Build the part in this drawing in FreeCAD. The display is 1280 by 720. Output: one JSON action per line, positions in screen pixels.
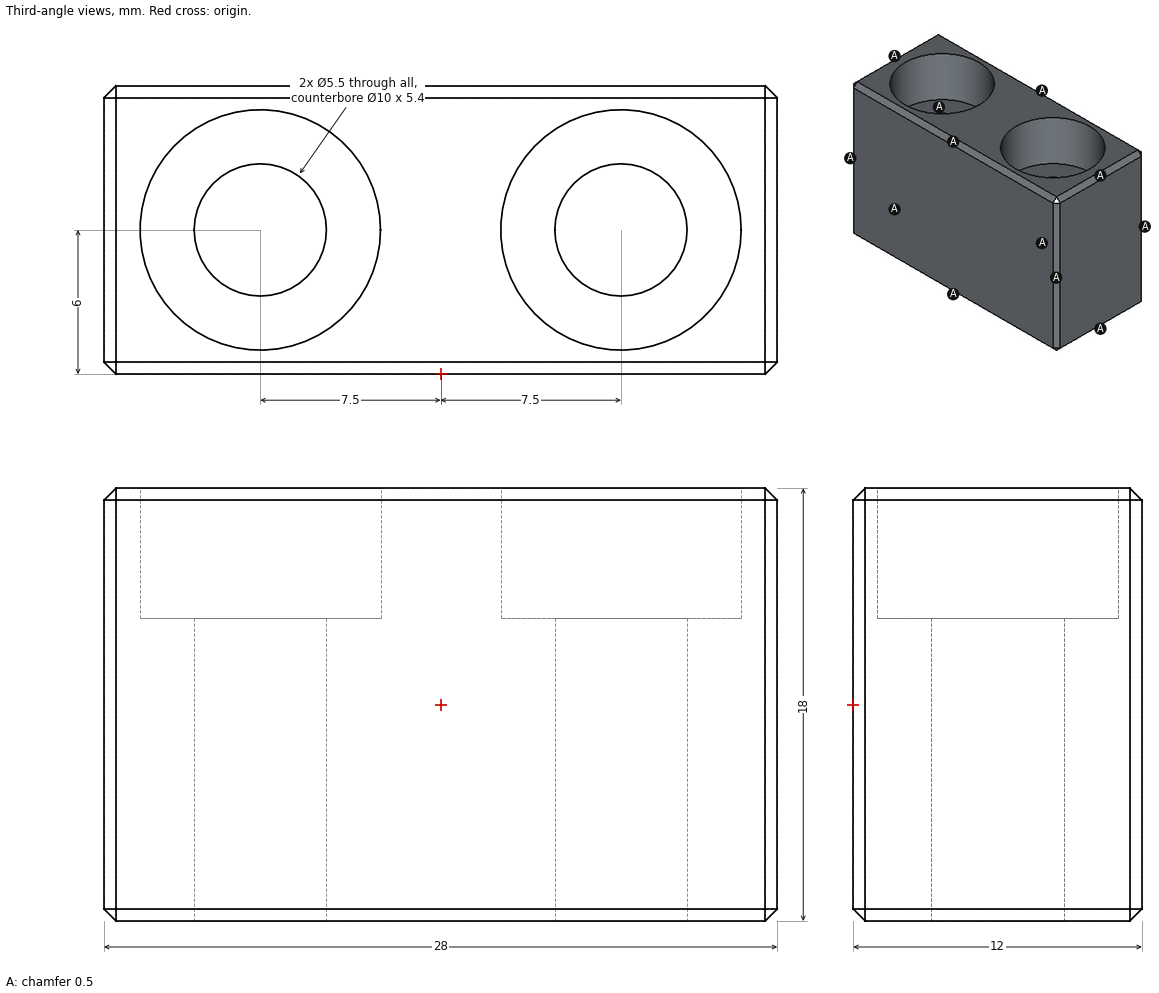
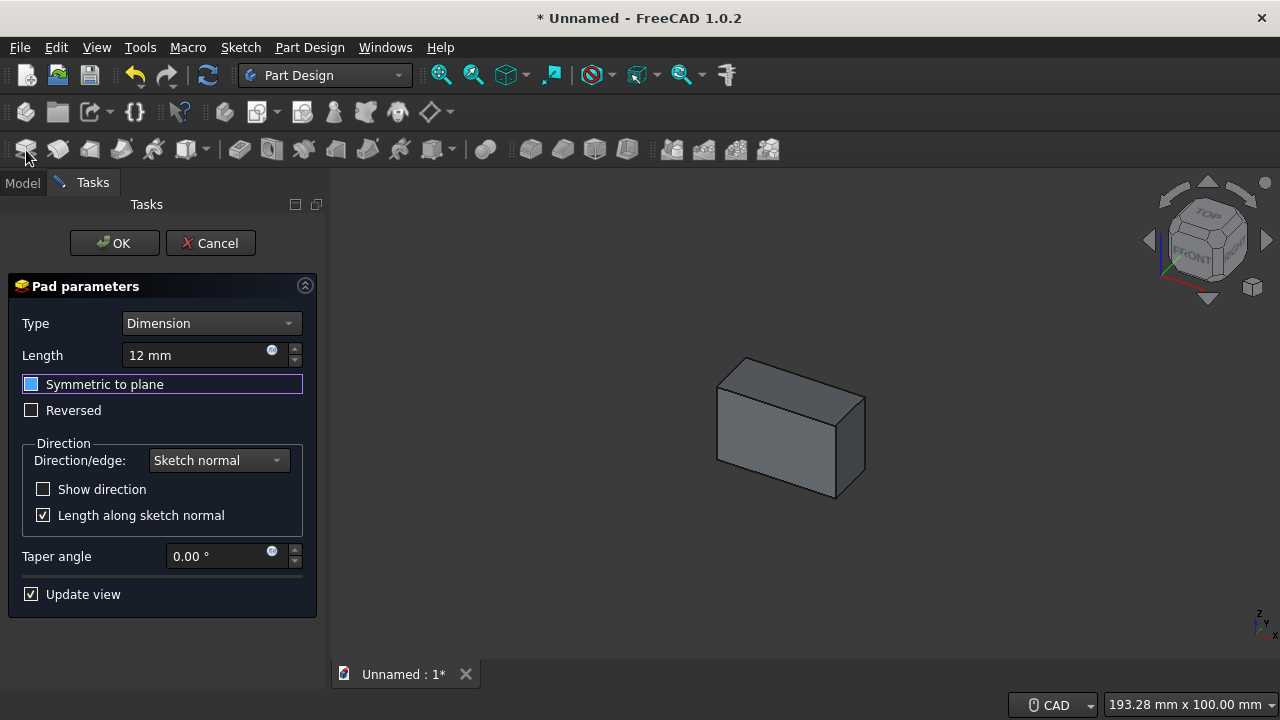
{"action": "left_click", "coordinate": [30, 410]}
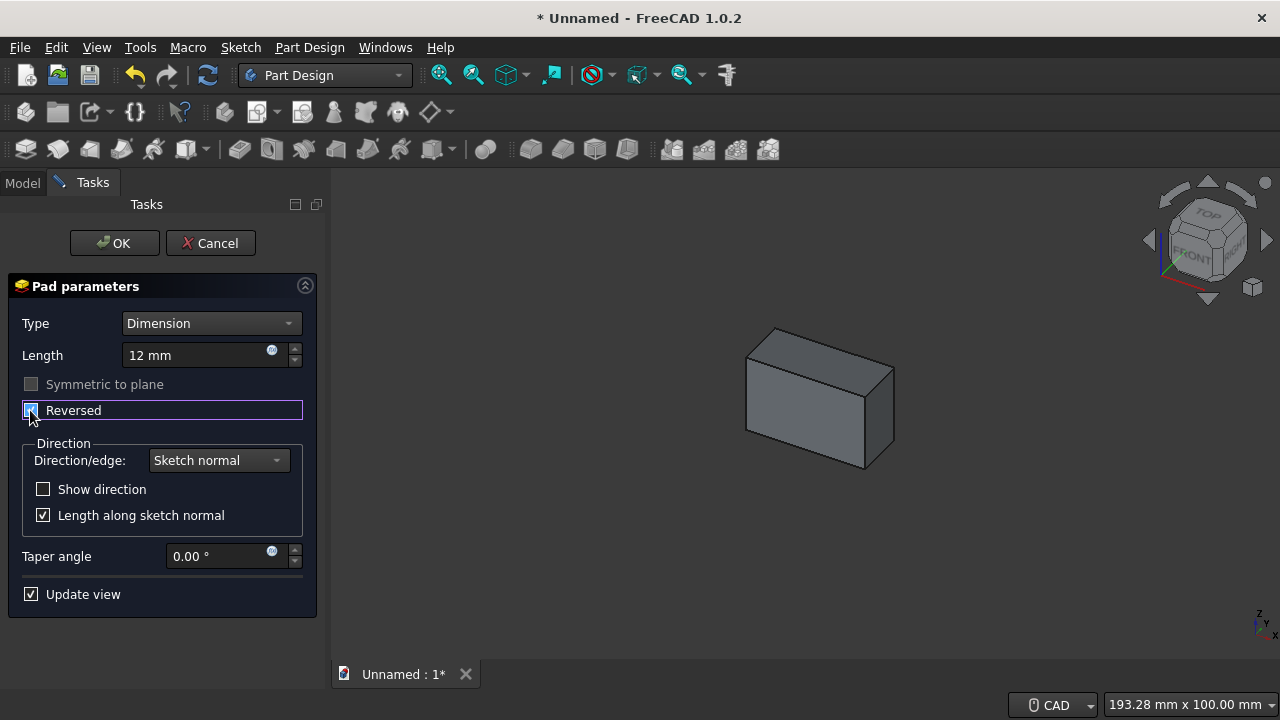
{"action": "left_click", "coordinate": [115, 243]}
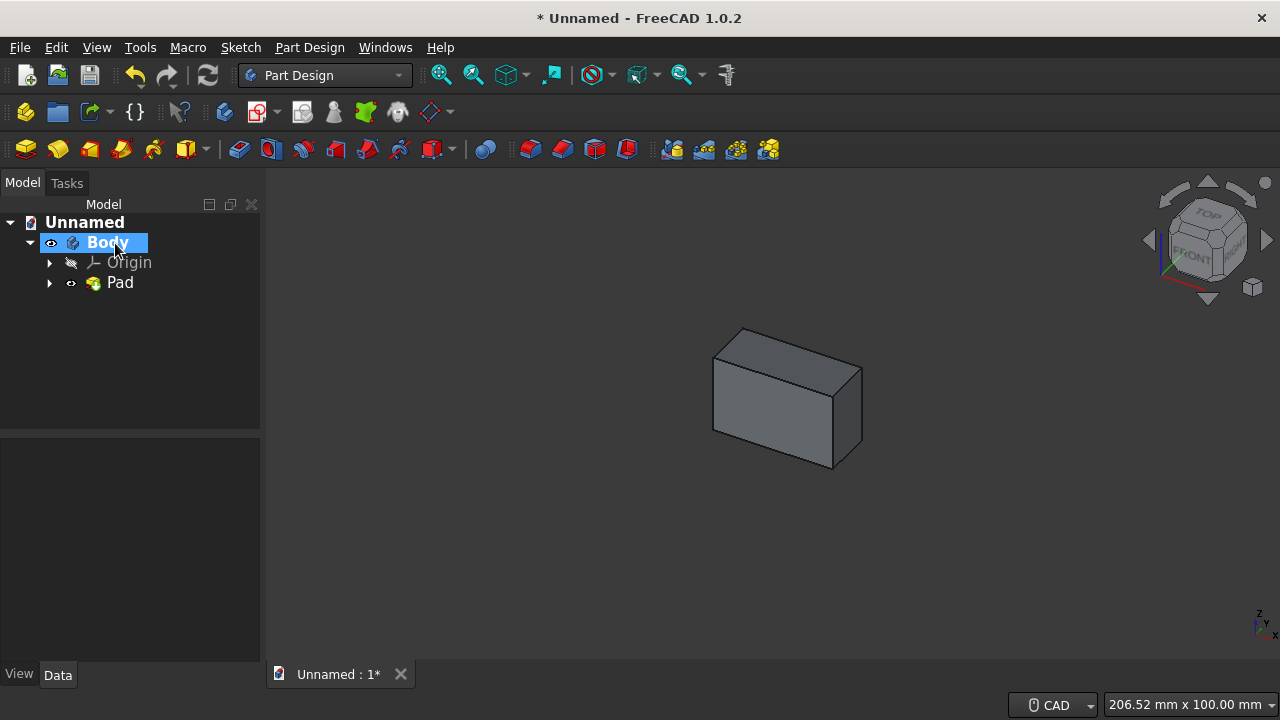
{"action": "left_click", "coordinate": [442, 76]}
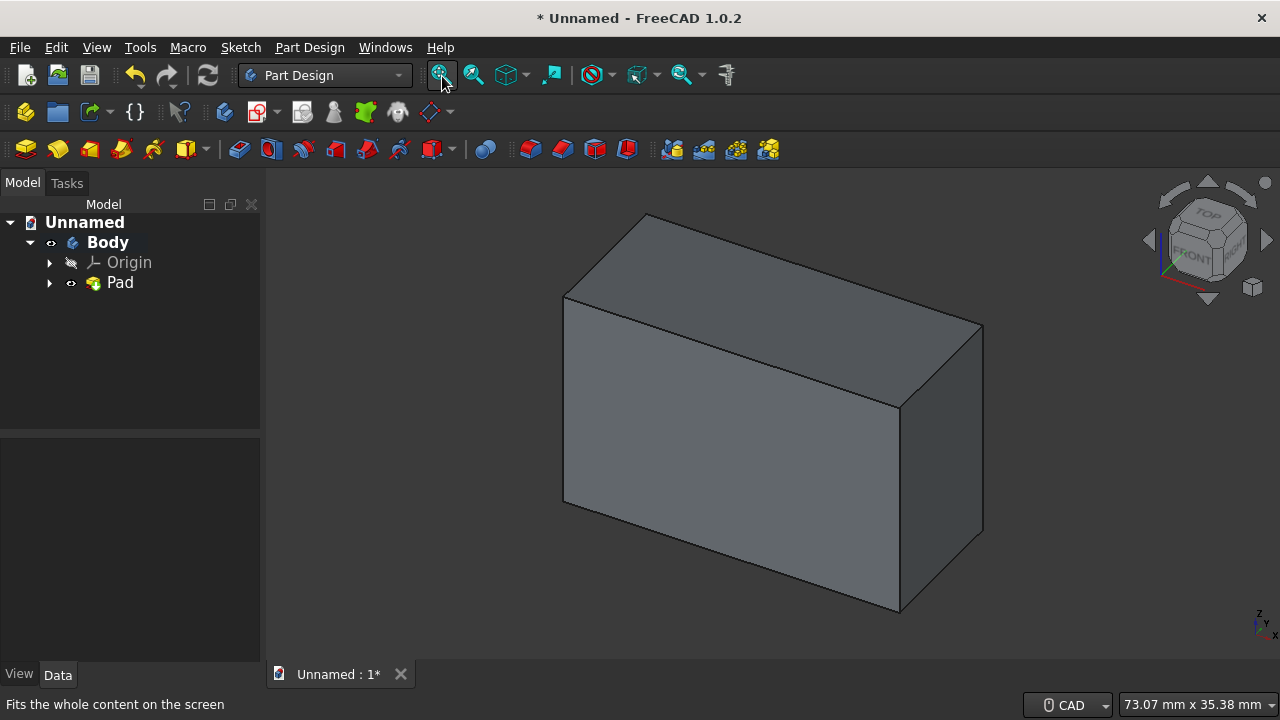
{"action": "left_click", "coordinate": [869, 342]}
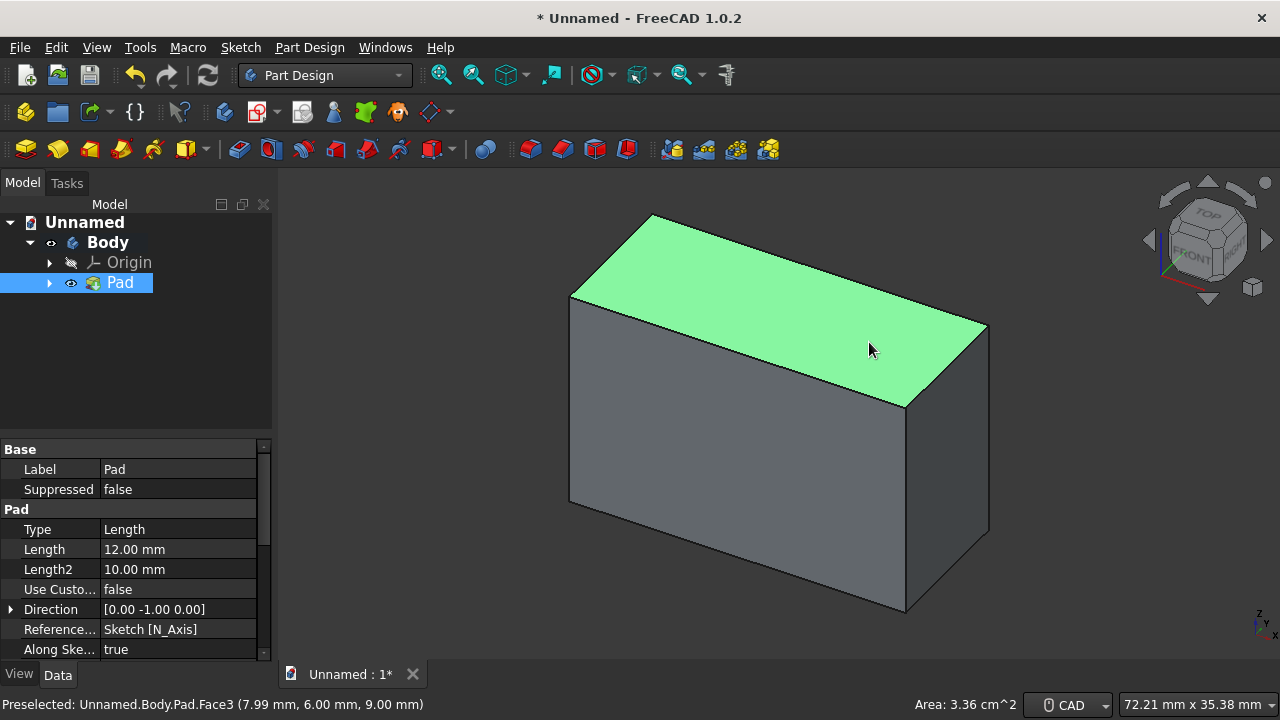
{"action": "left_click", "coordinate": [258, 112]}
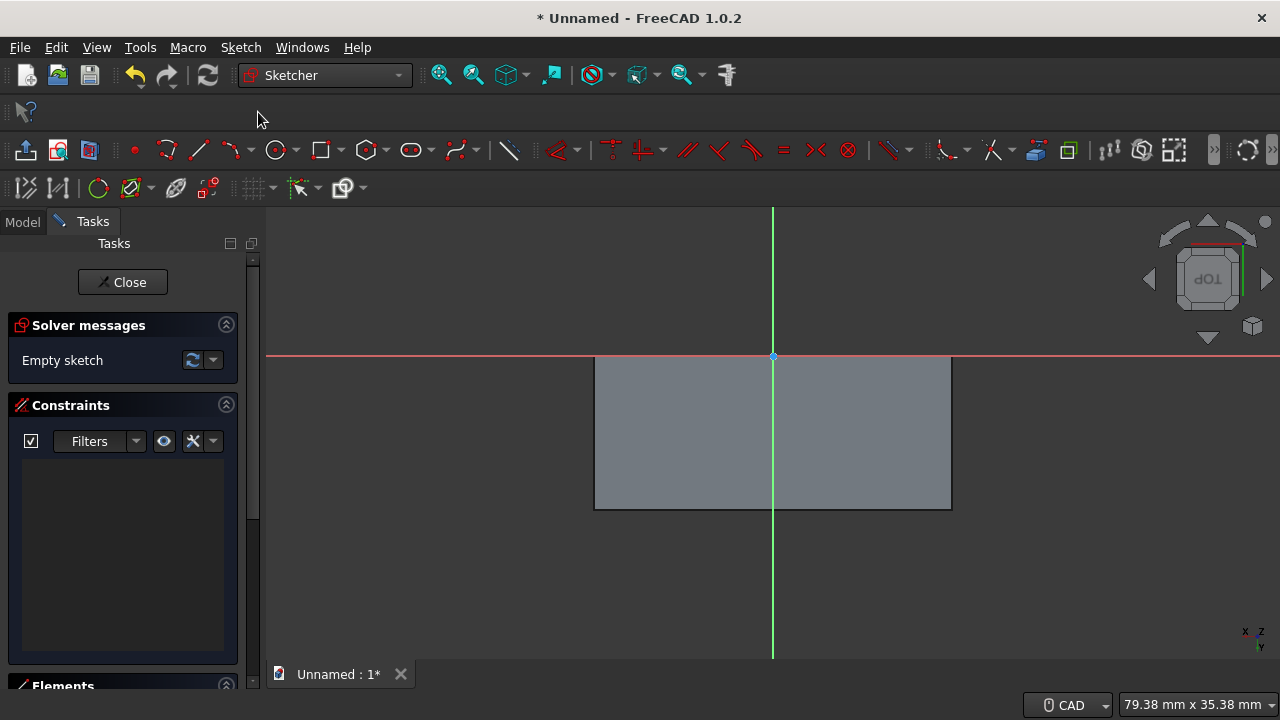
{"action": "scroll", "coordinate": [829, 395], "scroll_direction": "up", "scroll_amount": 4}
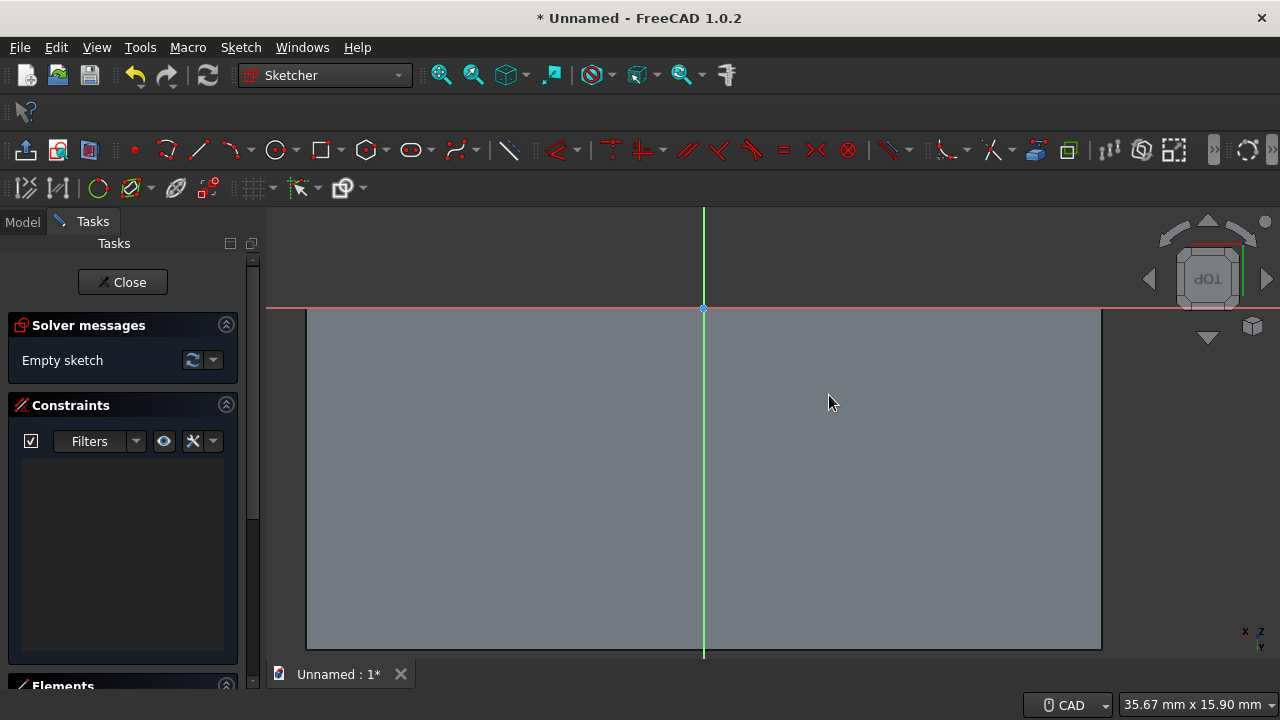
{"action": "key", "text": "g c"}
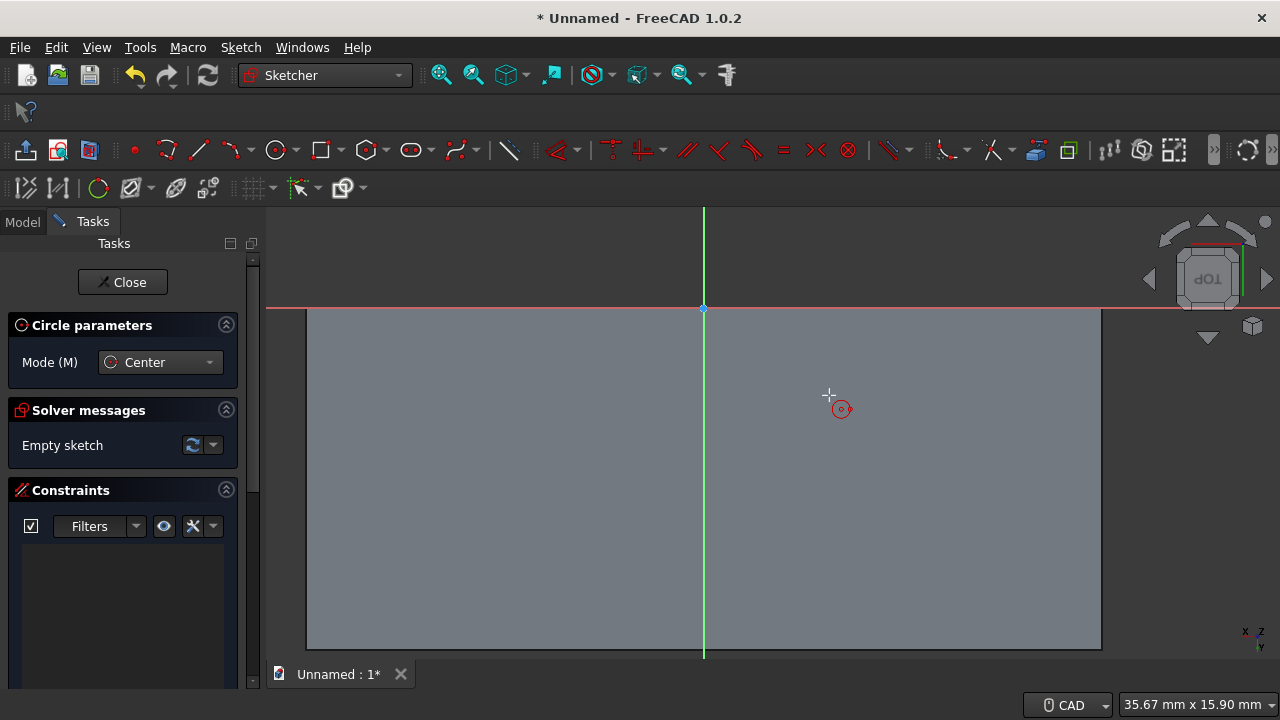
{"action": "left_click", "coordinate": [917, 479]}
{"action": "mouse_move", "coordinate": [972, 424]}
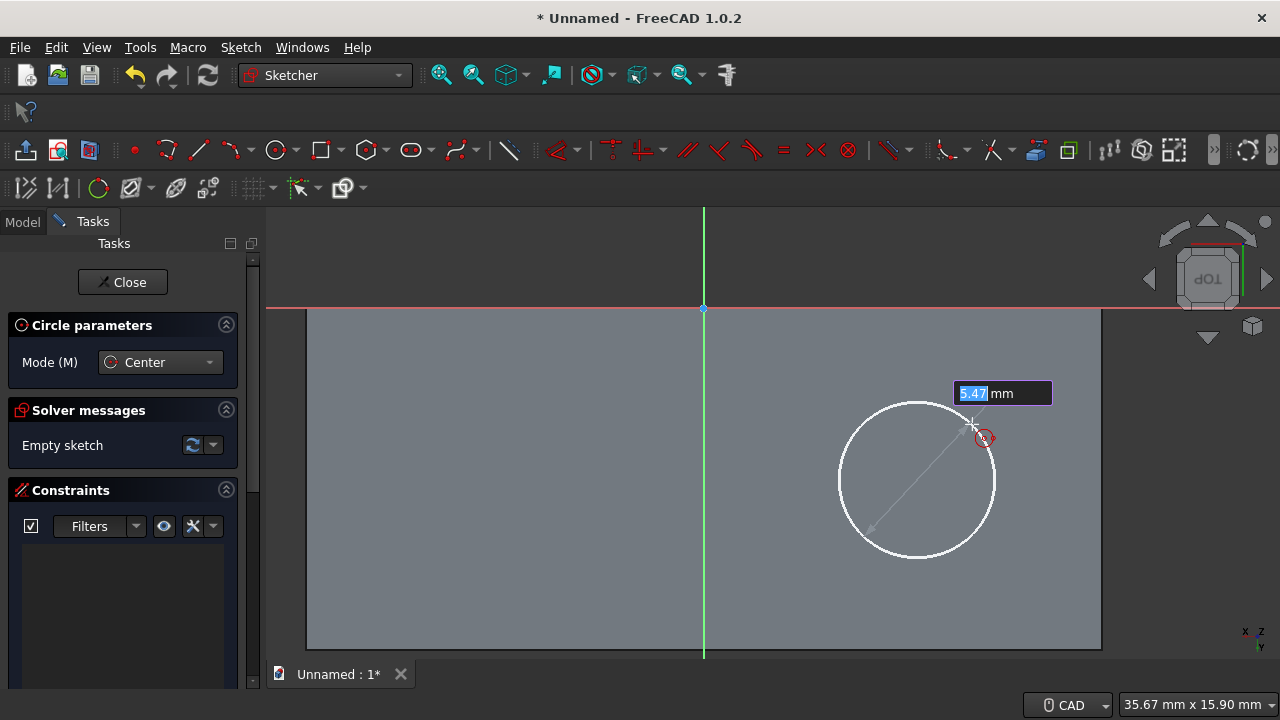
{"action": "type", "text": "5.5"}
{"action": "key", "text": "Return"}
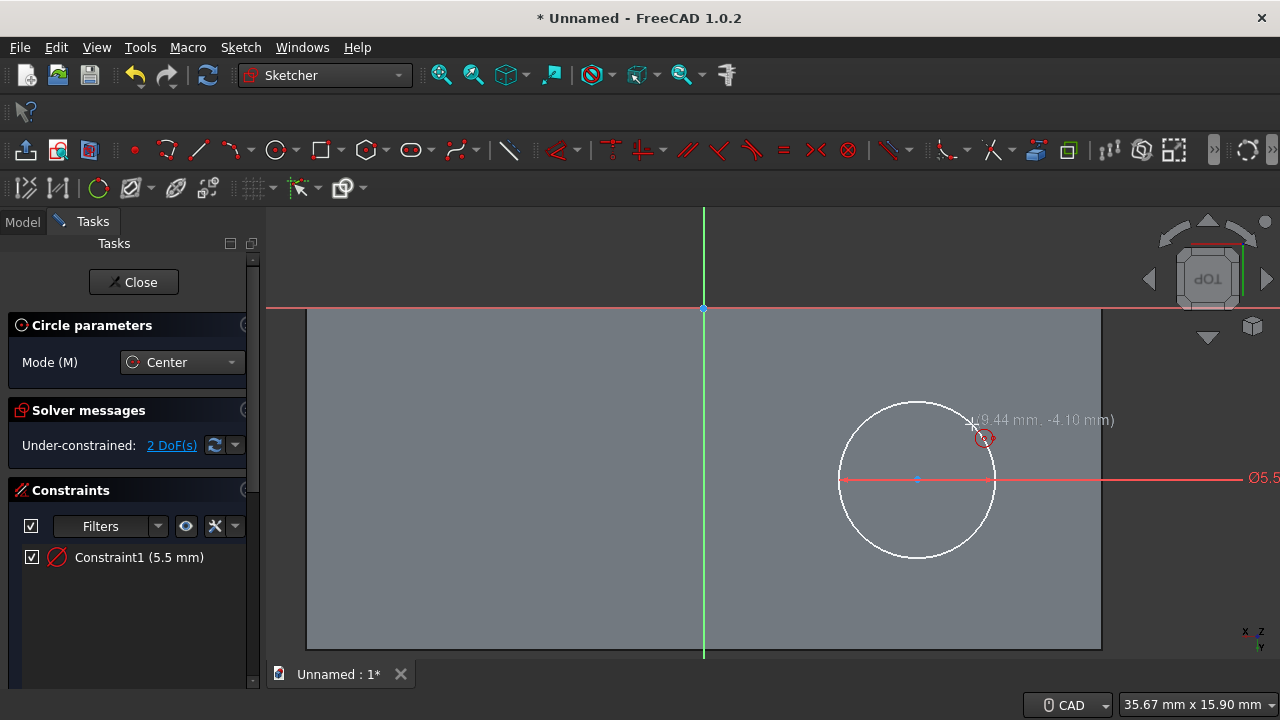
{"action": "left_click", "coordinate": [490, 479]}
{"action": "mouse_move", "coordinate": [546, 424]}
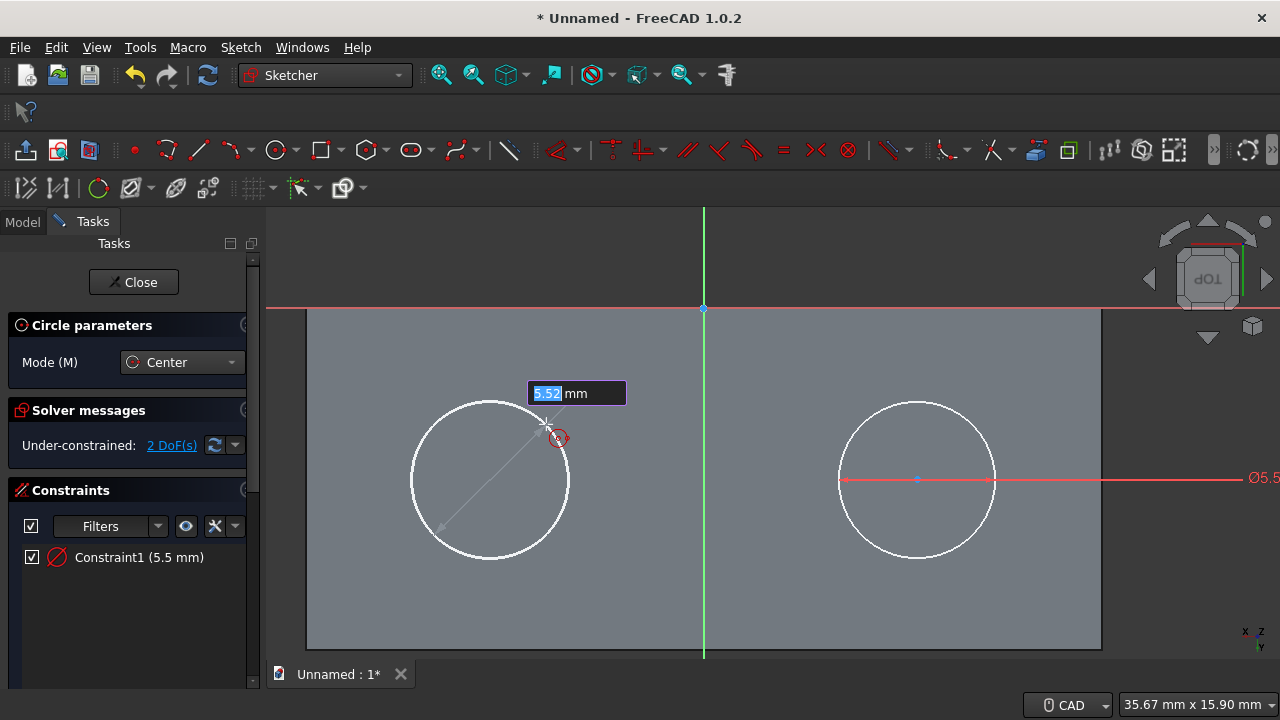
{"action": "type", "text": "5.5"}
{"action": "key", "text": "Return"}
{"action": "key", "text": "Escape"}